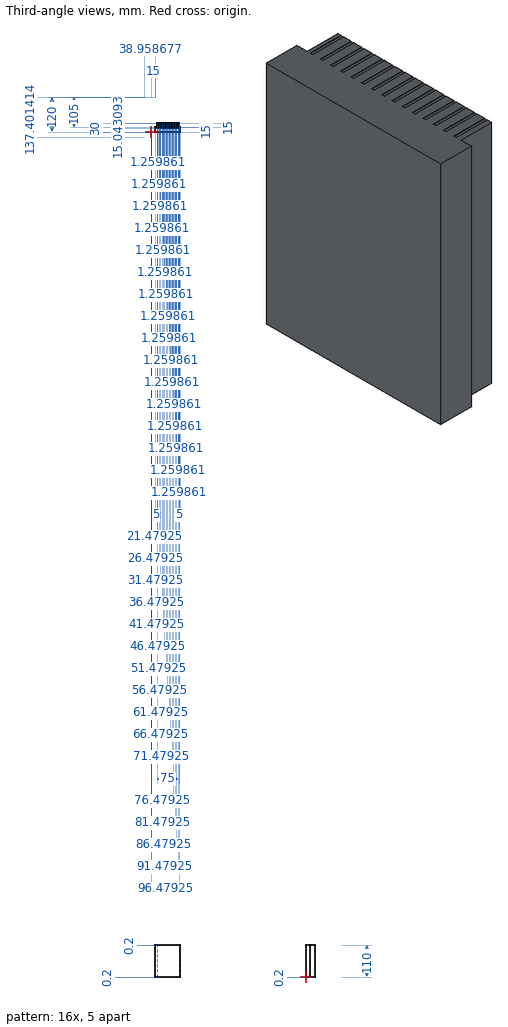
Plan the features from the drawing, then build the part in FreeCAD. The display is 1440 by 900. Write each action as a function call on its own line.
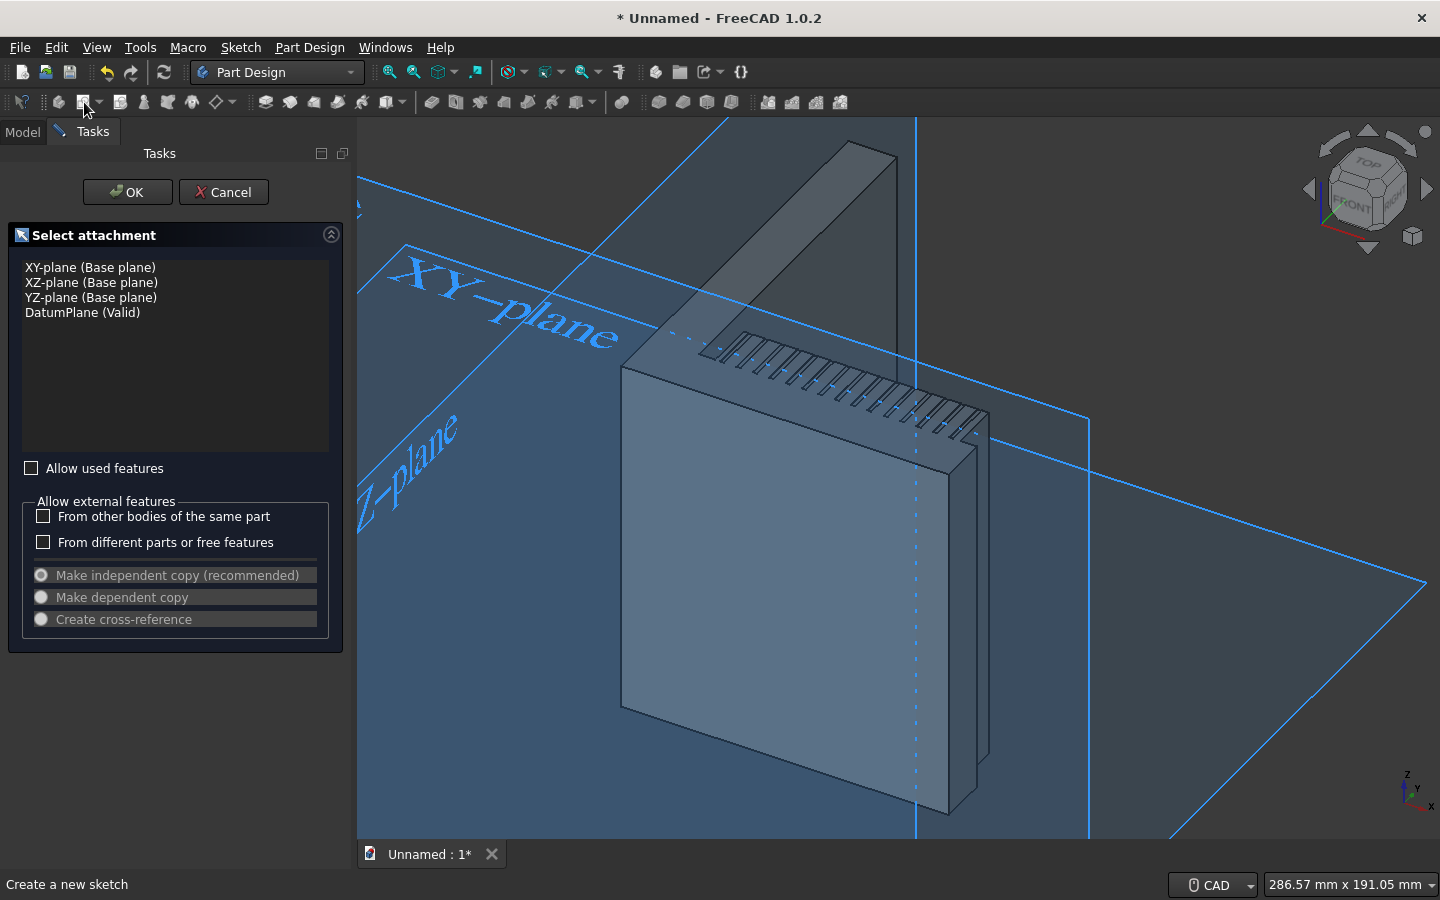
click(82, 268)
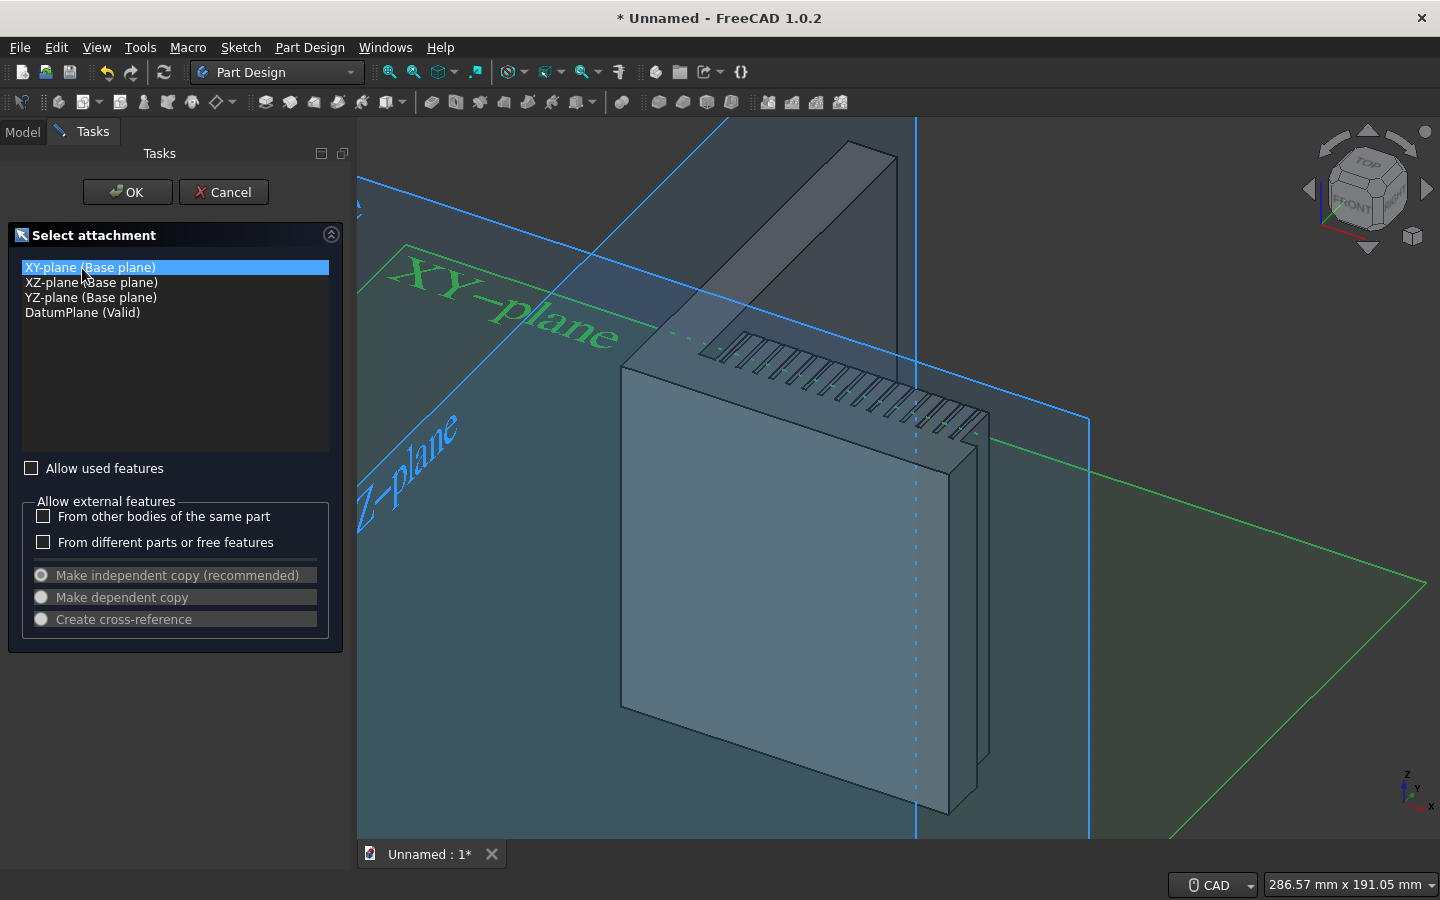
click(128, 192)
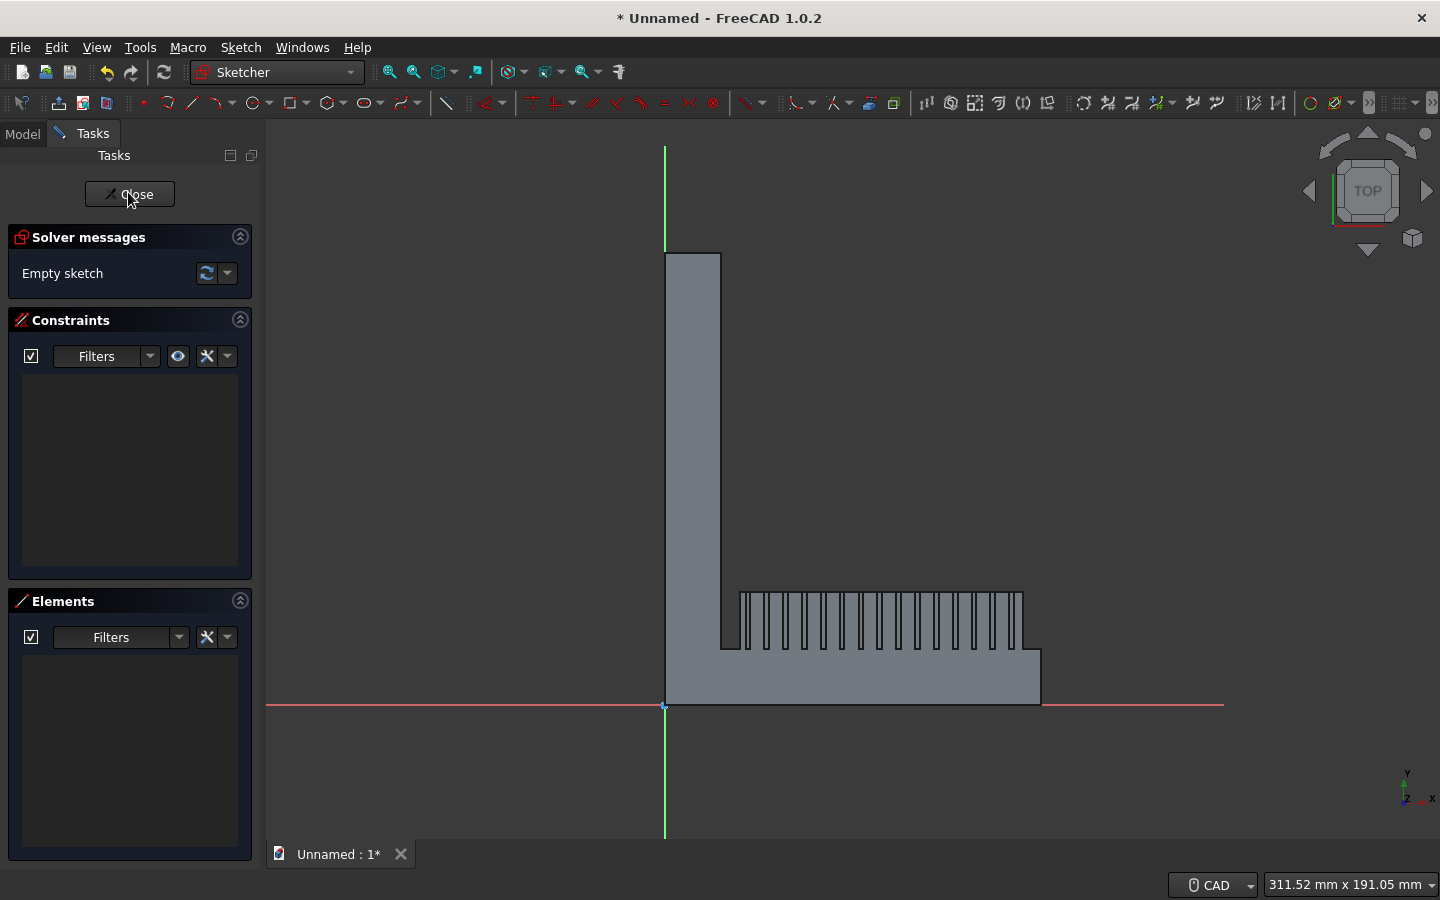
key(q)
key(s)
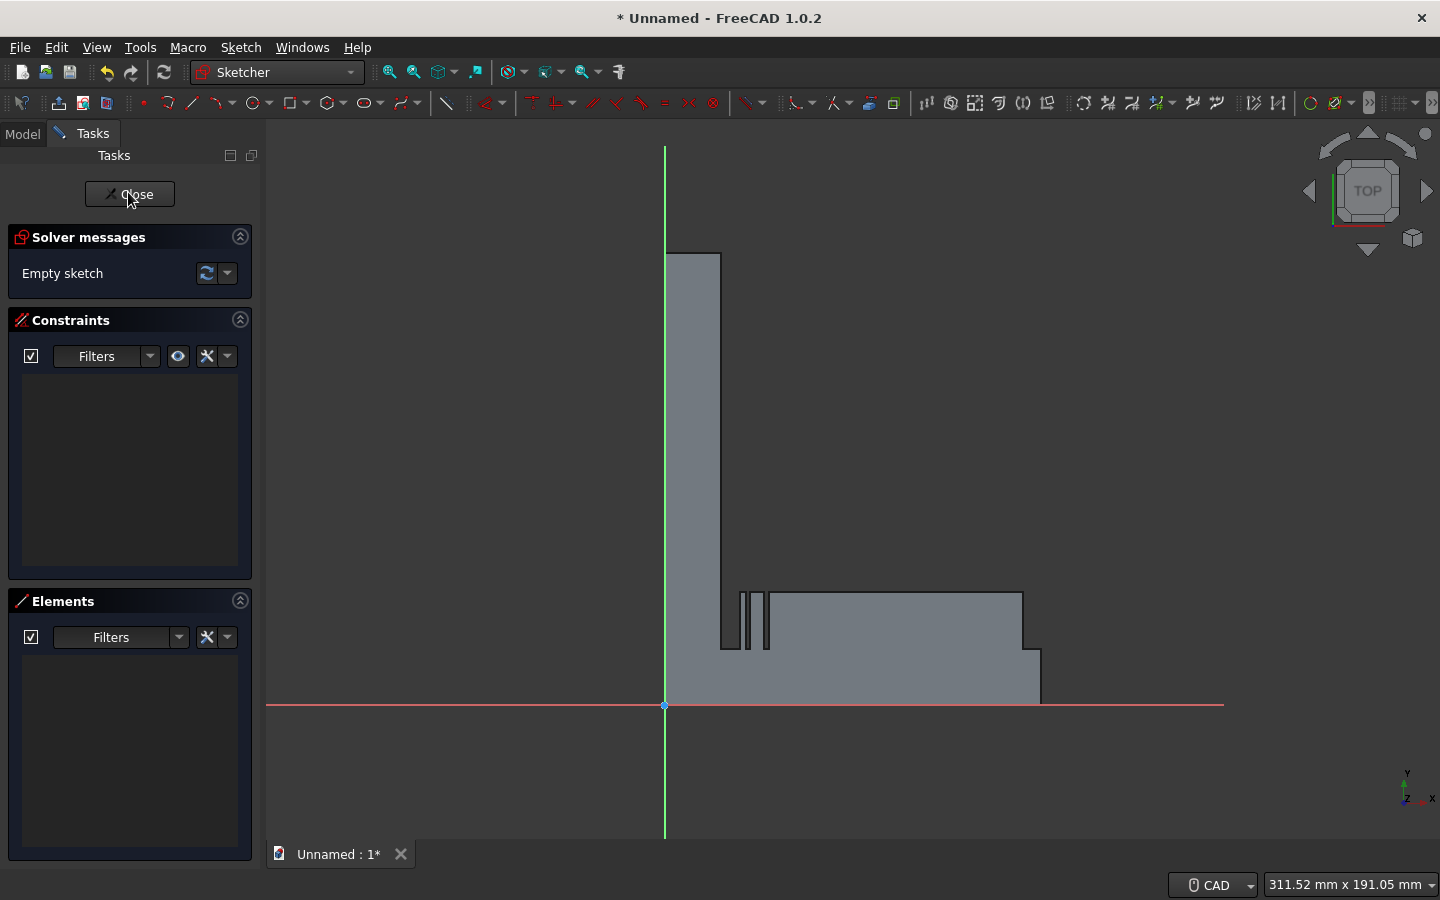
scroll(707, 704, up, 7)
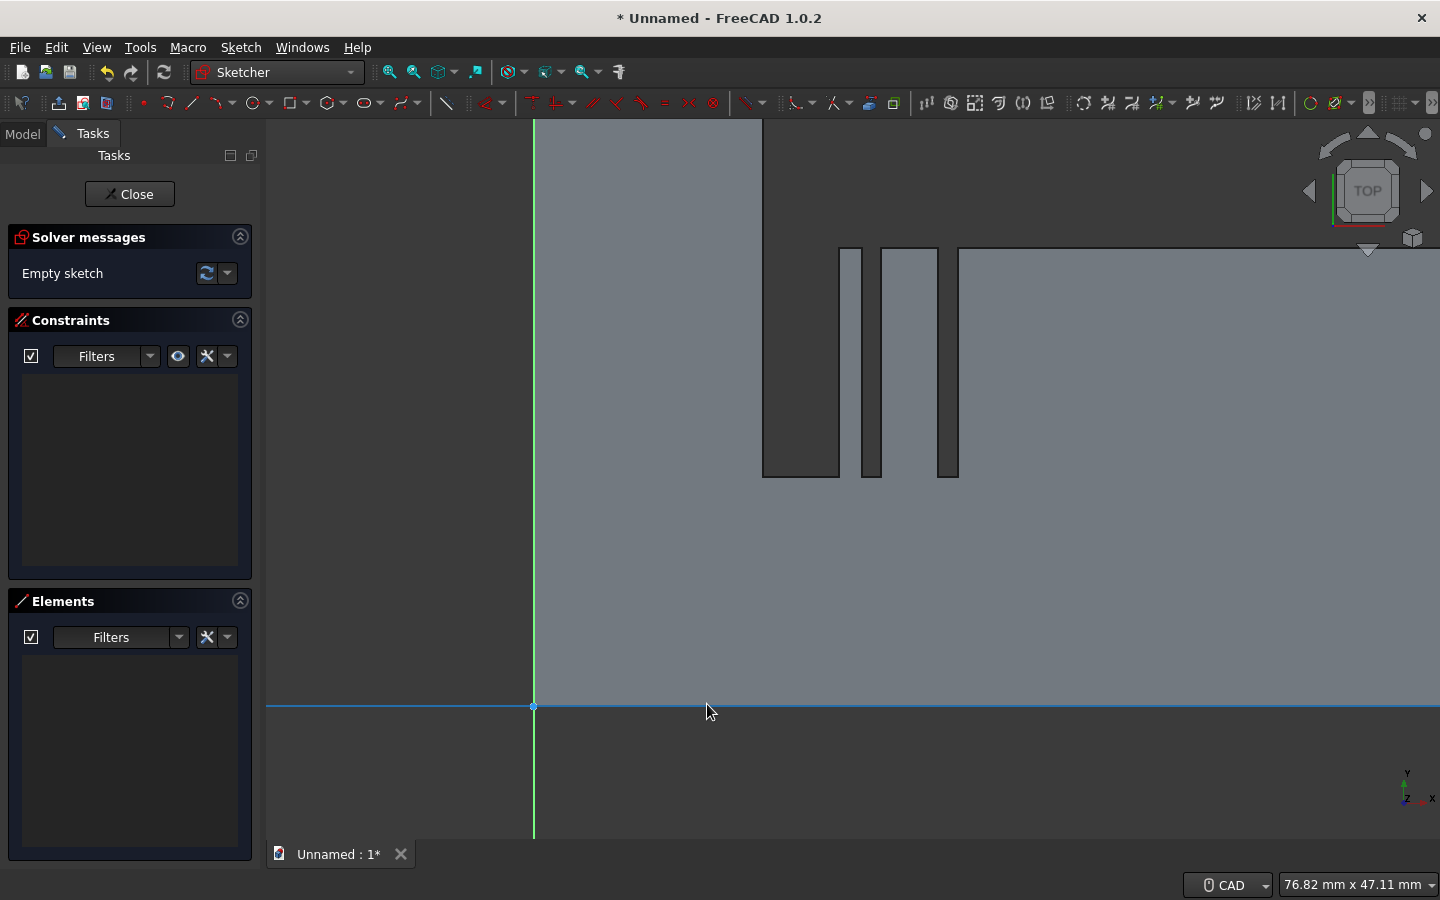
key(g)
key(r)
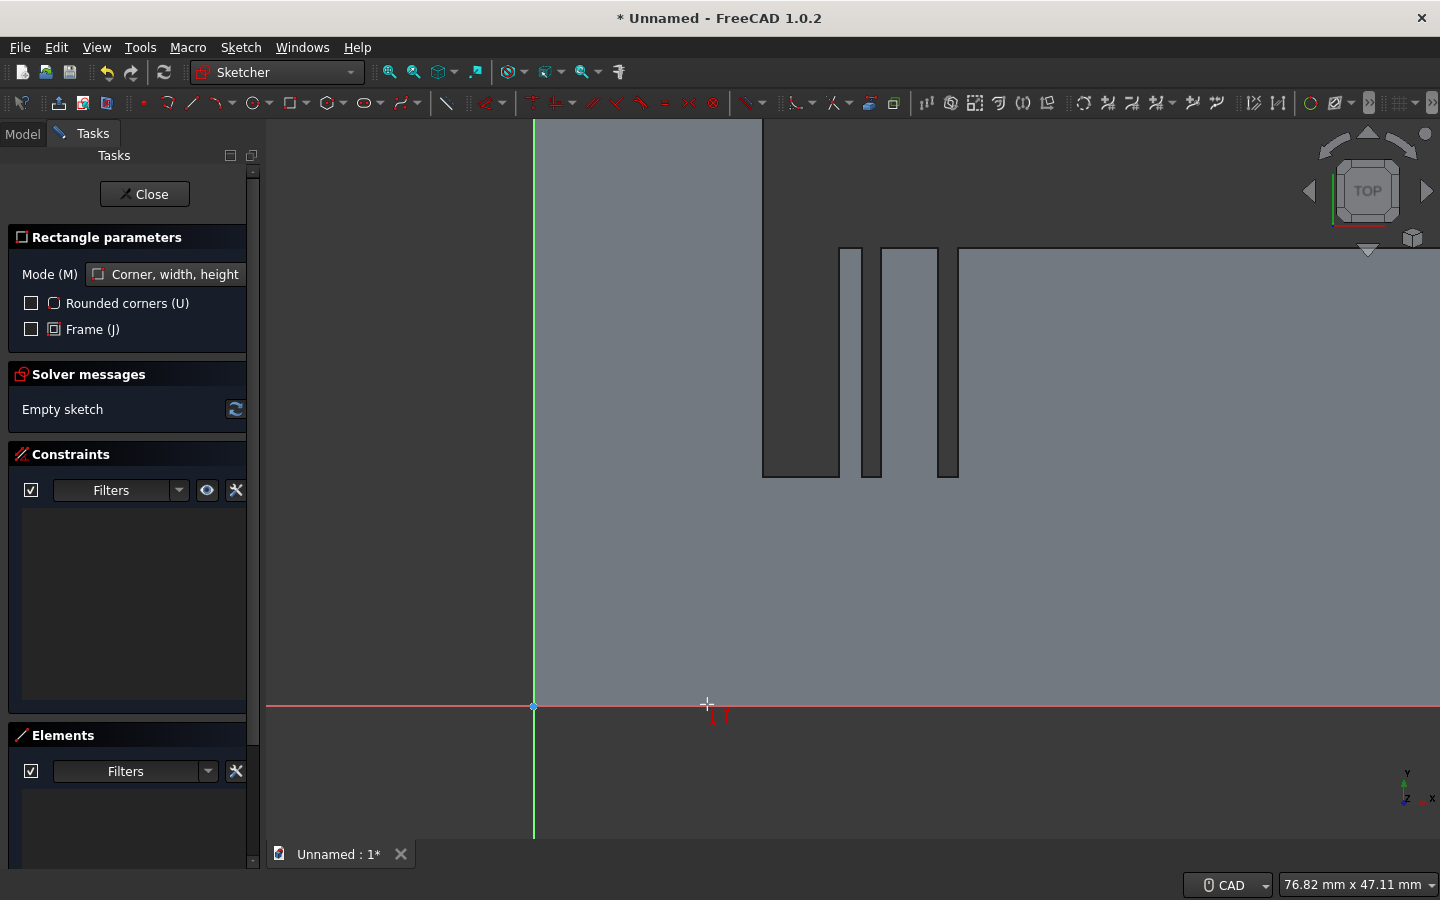
click(1015, 248)
click(1034, 477)
key(Escape)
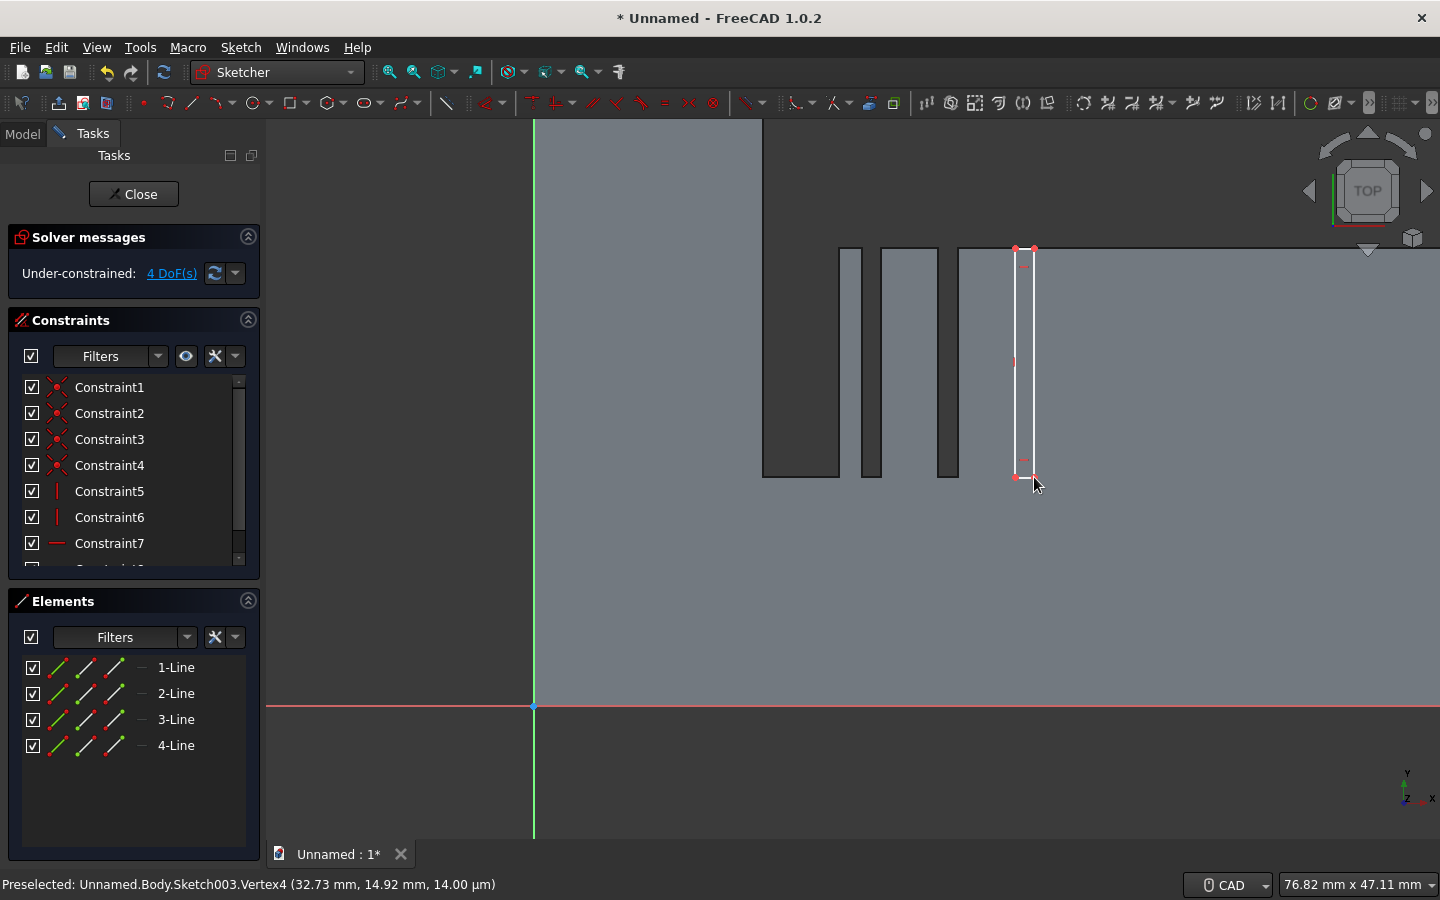
click(486, 104)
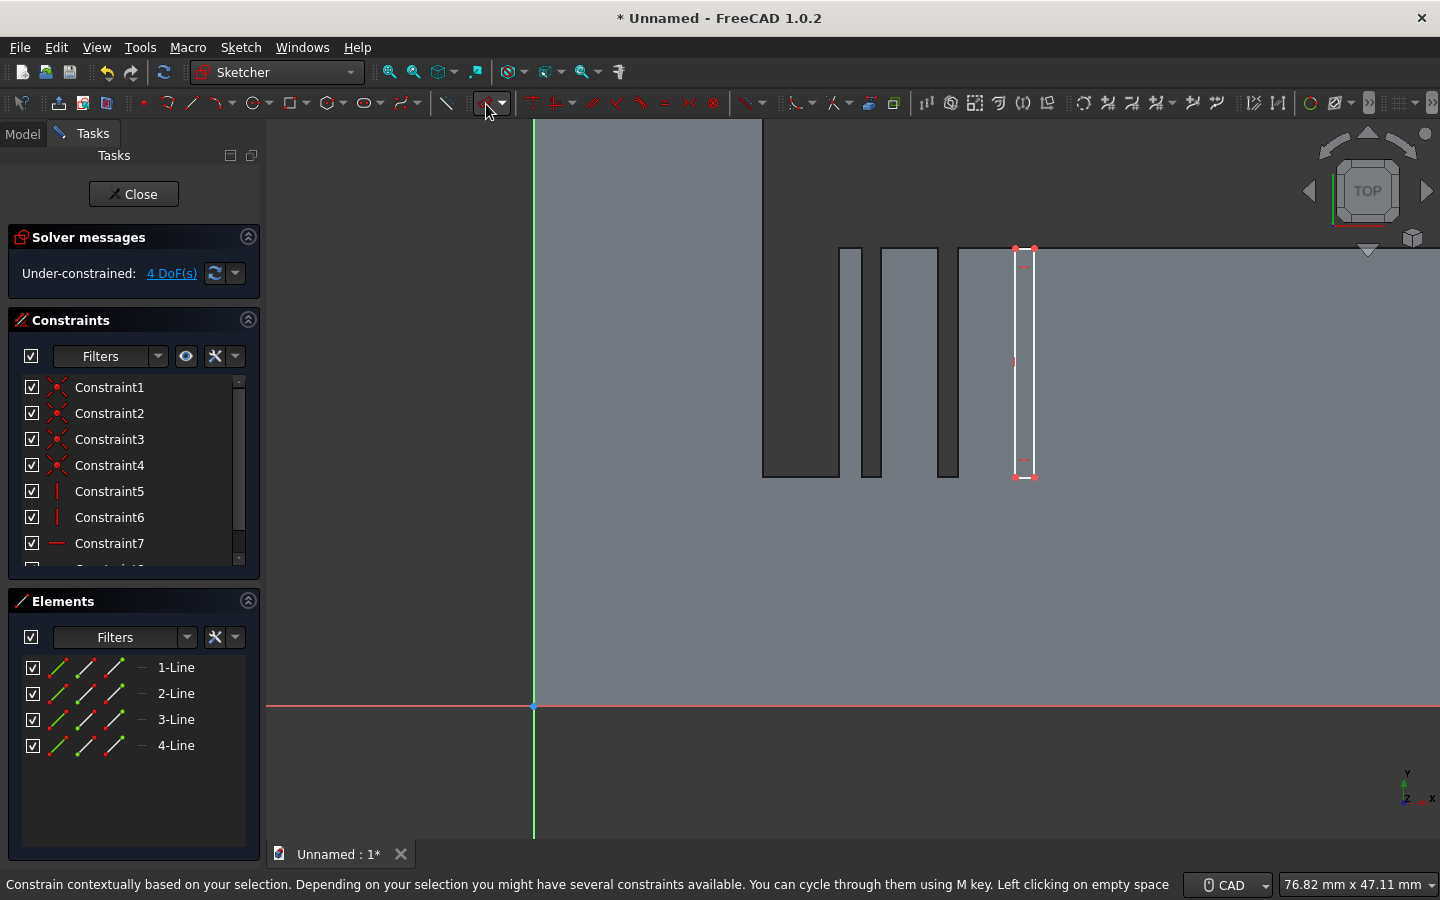
click(1015, 249)
click(500, 478)